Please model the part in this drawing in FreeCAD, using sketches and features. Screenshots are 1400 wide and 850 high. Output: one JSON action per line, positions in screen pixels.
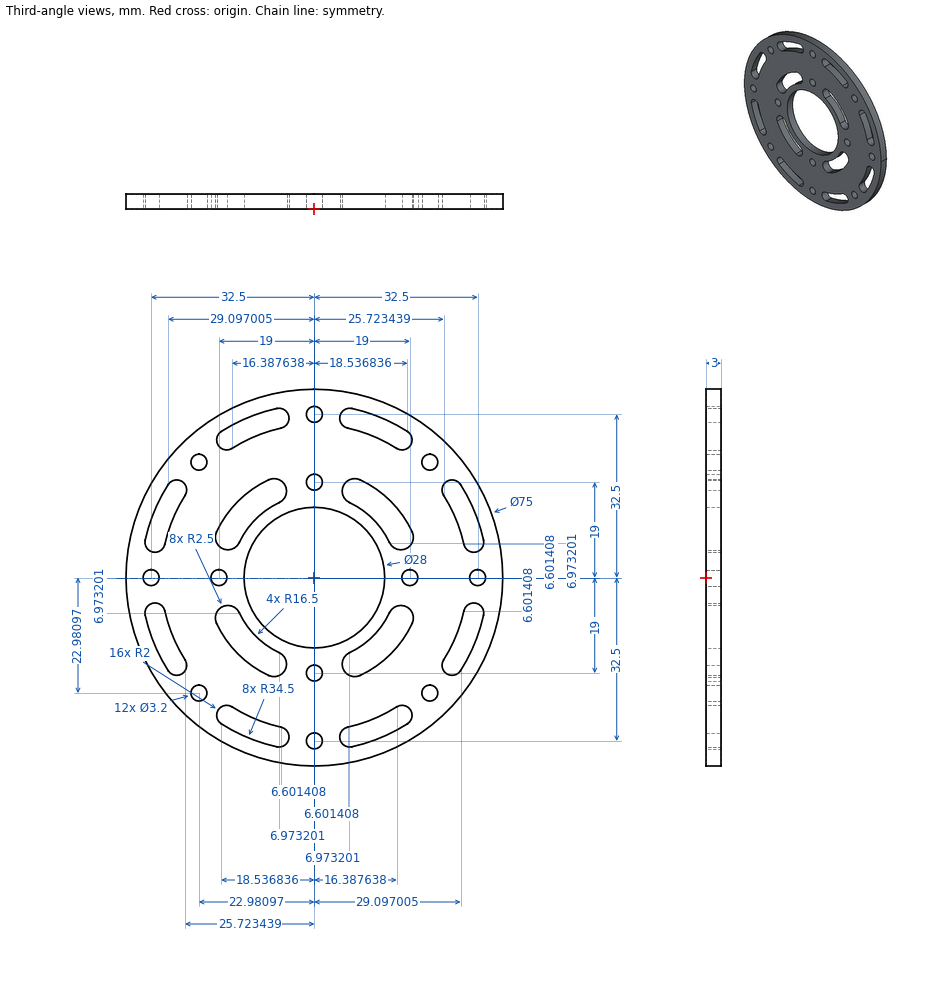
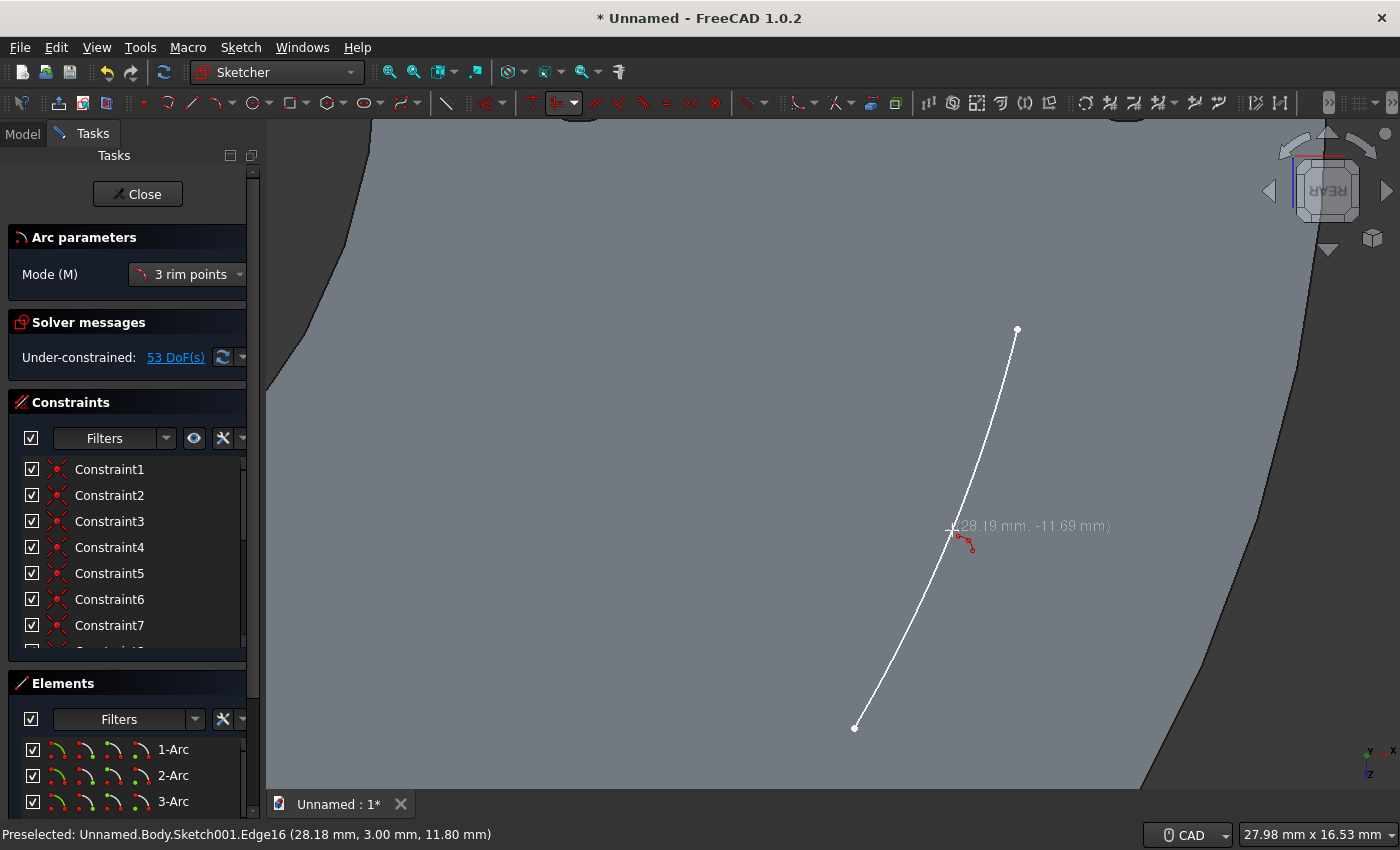
{"action": "scroll", "coordinate": [954, 533], "scroll_direction": "down", "scroll_amount": 9}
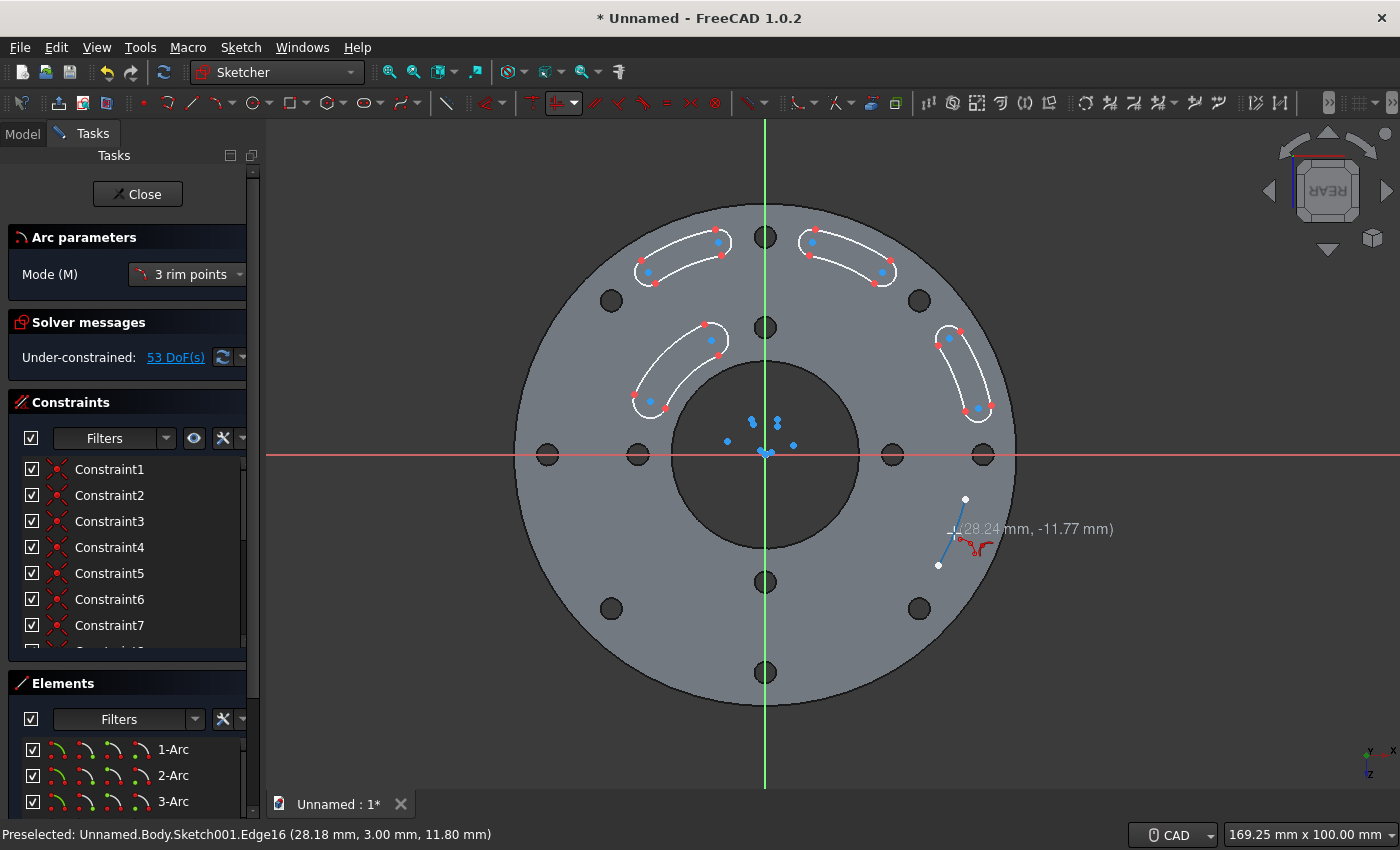
{"action": "left_click", "coordinate": [938, 566]}
{"action": "left_click", "coordinate": [960, 579]}
{"action": "left_click", "coordinate": [942, 583]}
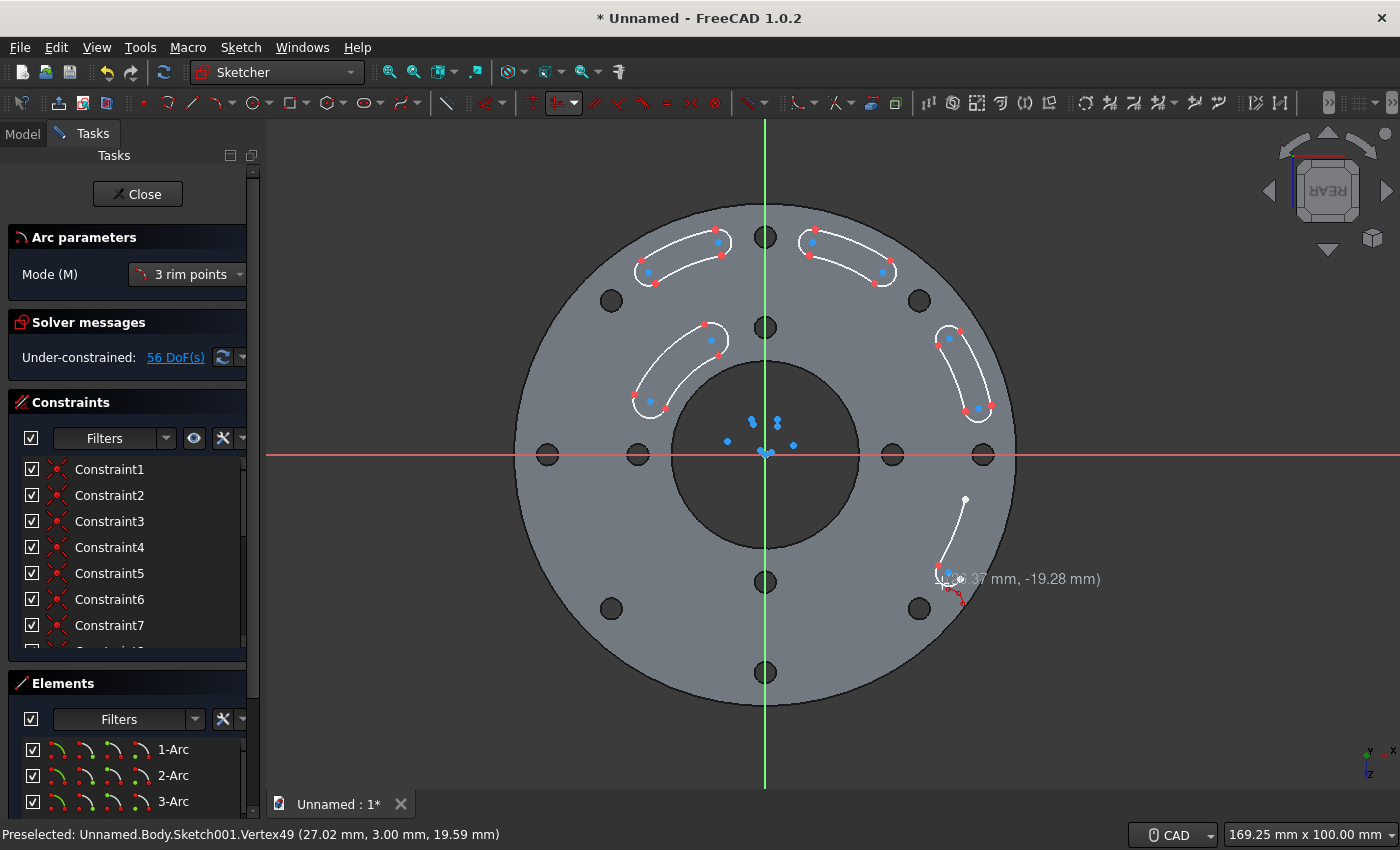
{"action": "left_click", "coordinate": [960, 580]}
{"action": "left_click", "coordinate": [991, 505]}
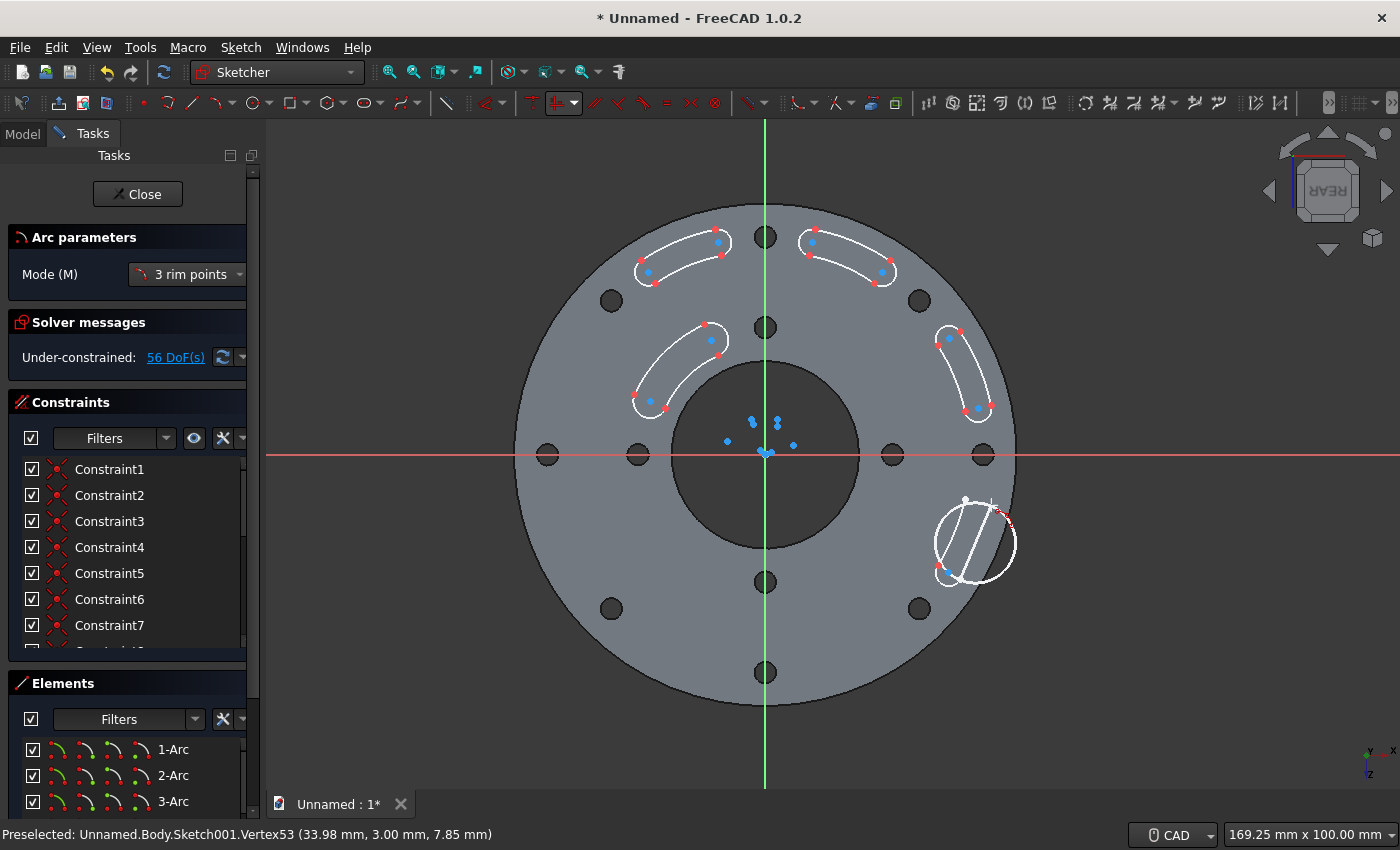
{"action": "scroll", "coordinate": [979, 543], "scroll_direction": "up", "scroll_amount": 8}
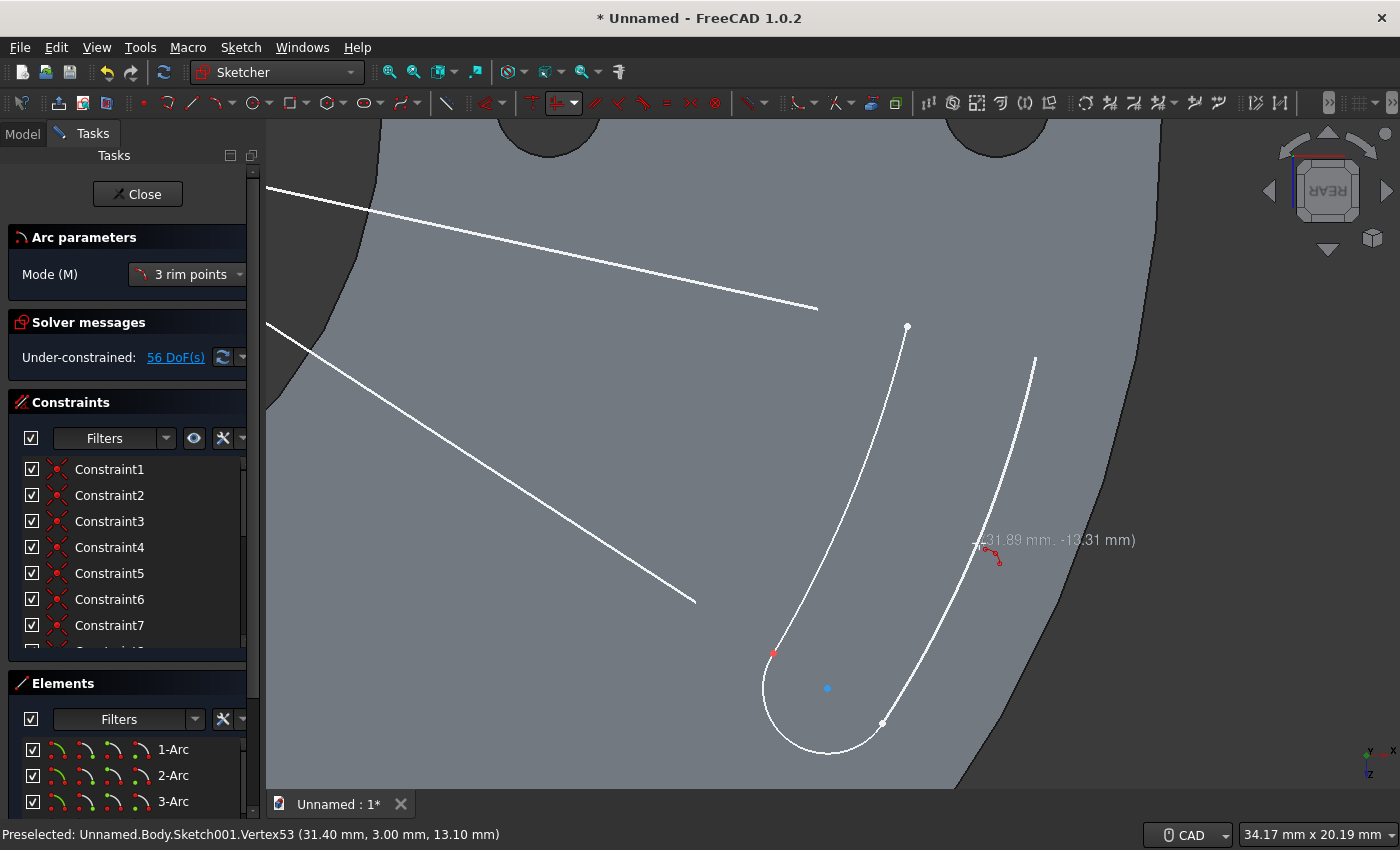
{"action": "left_click", "coordinate": [976, 542]}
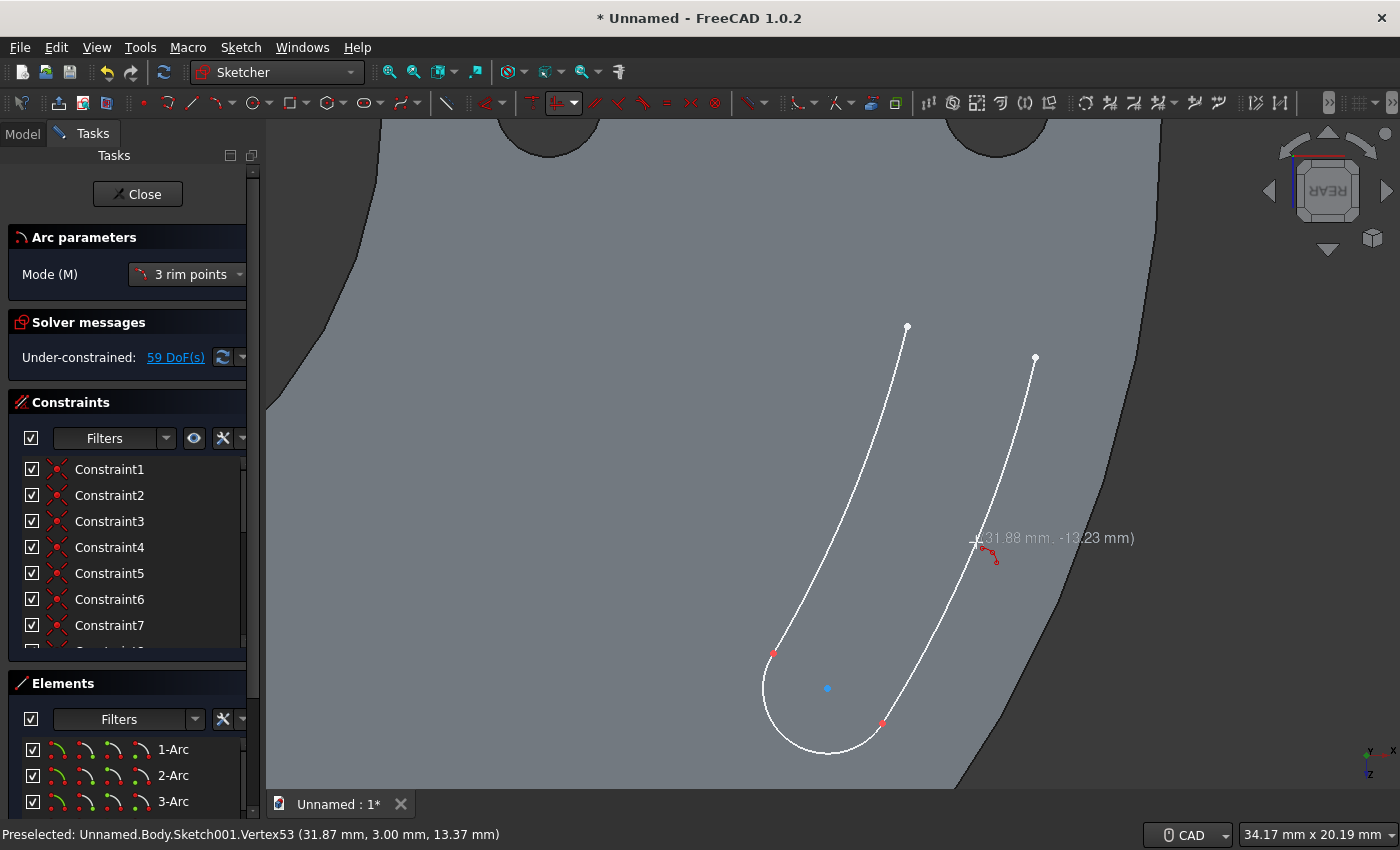
{"action": "scroll", "coordinate": [979, 543], "scroll_direction": "down", "scroll_amount": 8}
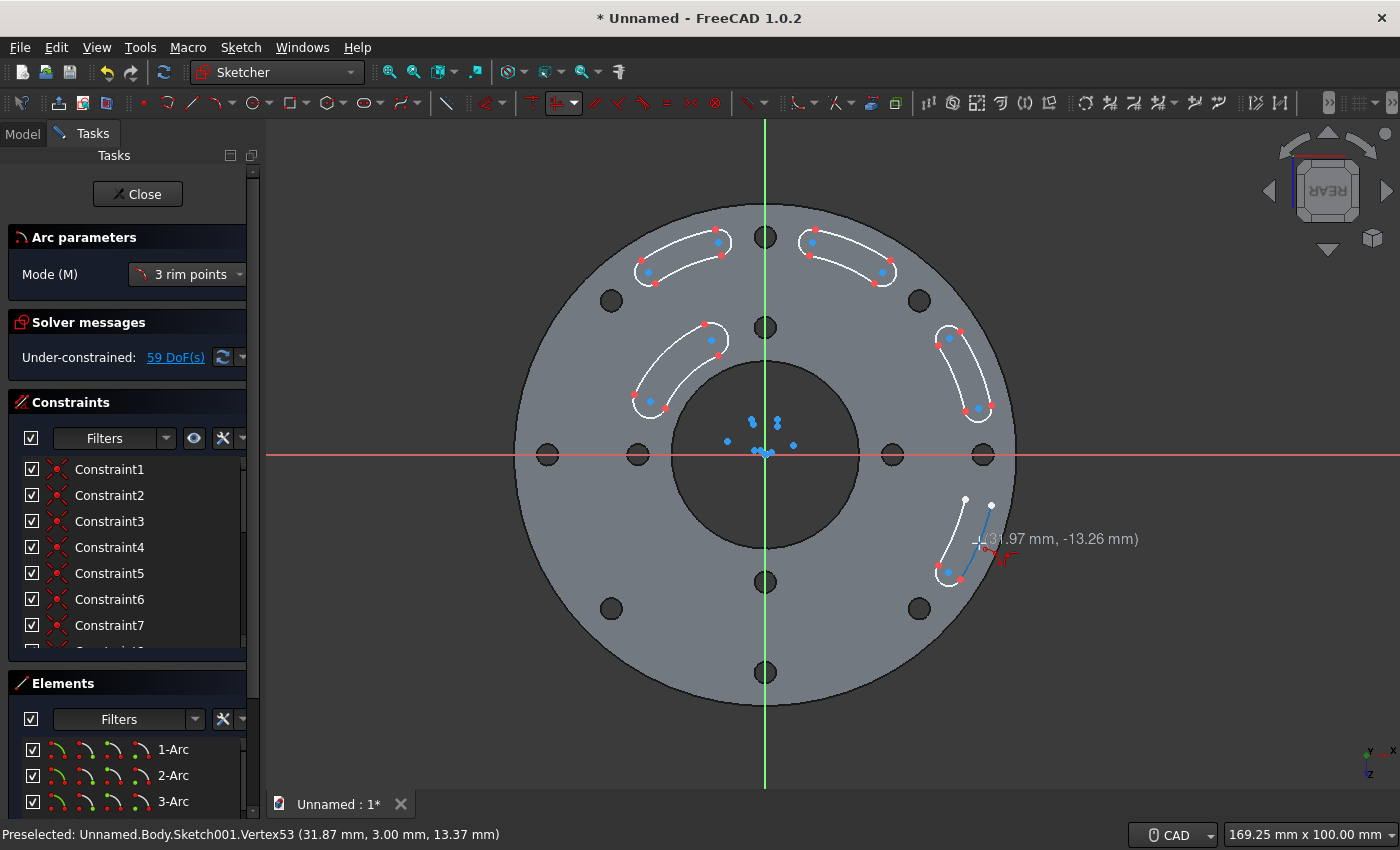
{"action": "left_click", "coordinate": [991, 506]}
{"action": "left_click", "coordinate": [965, 500]}
{"action": "left_click", "coordinate": [981, 489]}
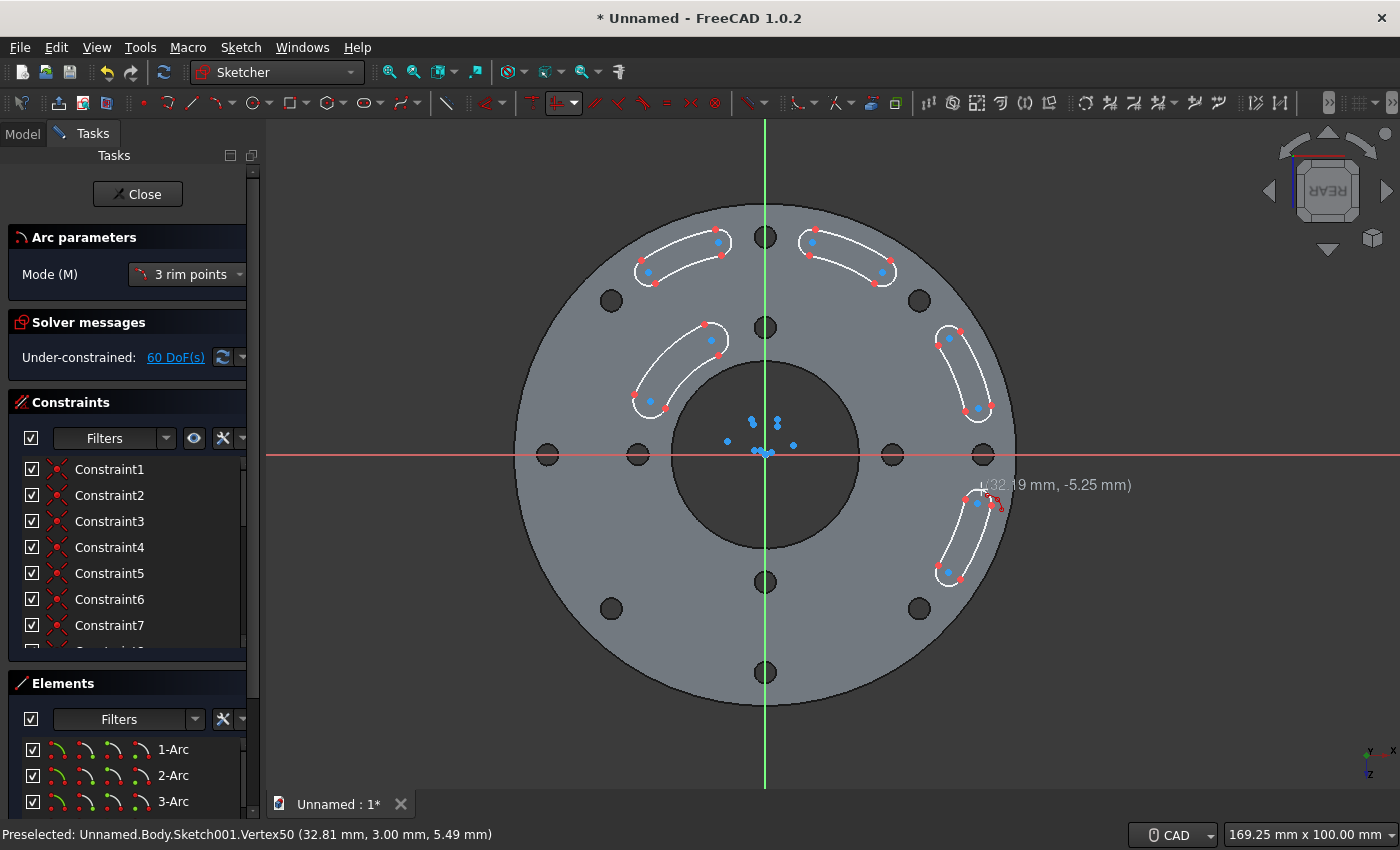
{"action": "left_click", "coordinate": [810, 654]}
{"action": "left_click", "coordinate": [815, 681]}
{"action": "left_click", "coordinate": [799, 670]}